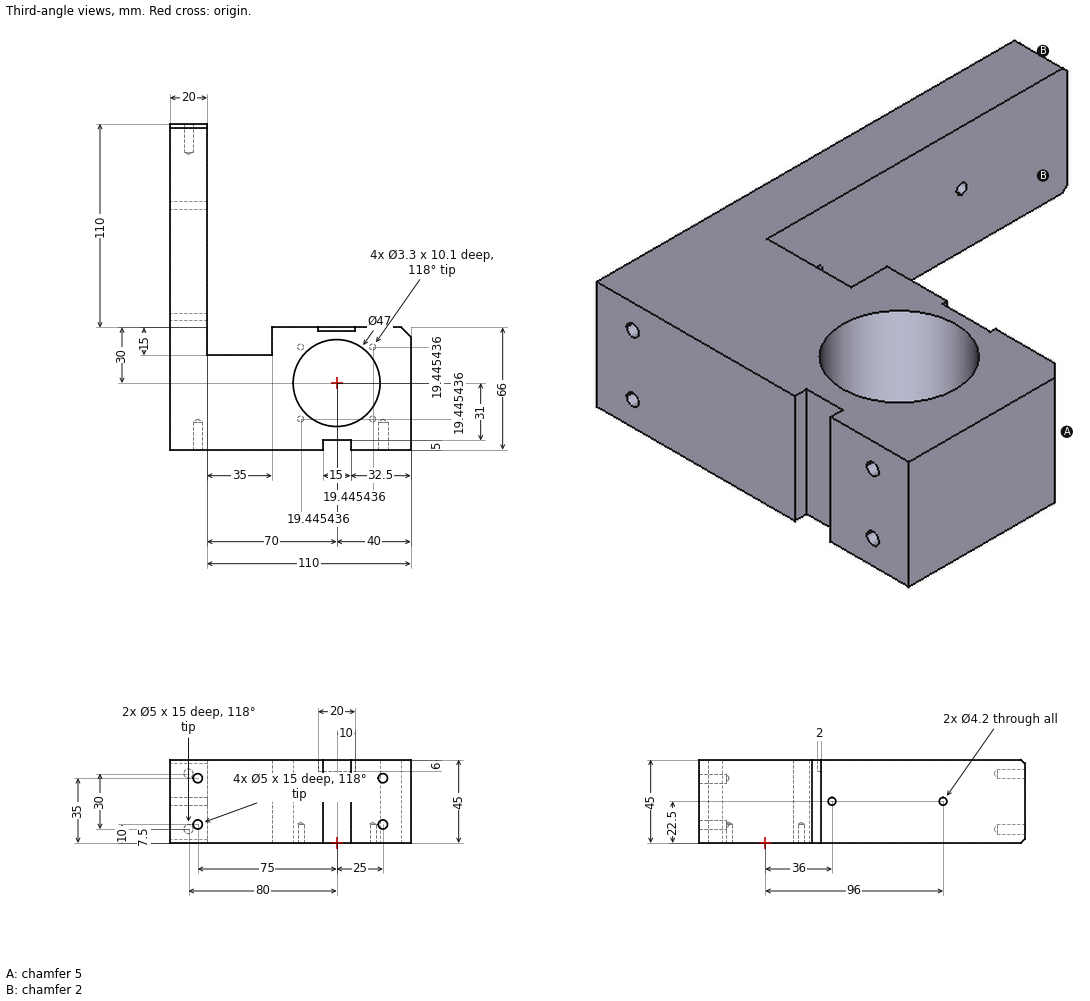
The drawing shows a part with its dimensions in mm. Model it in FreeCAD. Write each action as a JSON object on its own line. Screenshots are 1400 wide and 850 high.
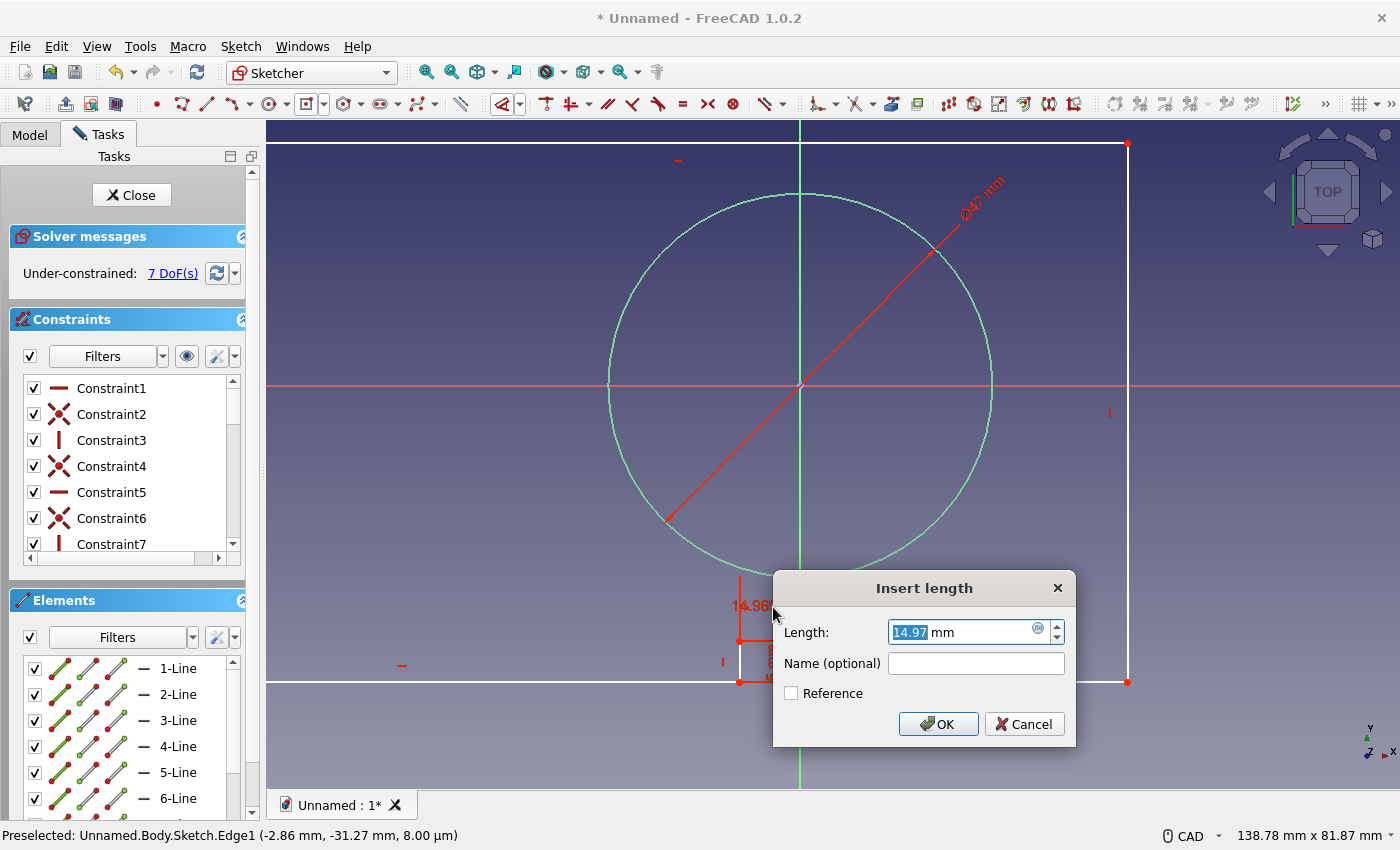
{"action": "type", "text": "15"}
{"action": "key", "text": "Return"}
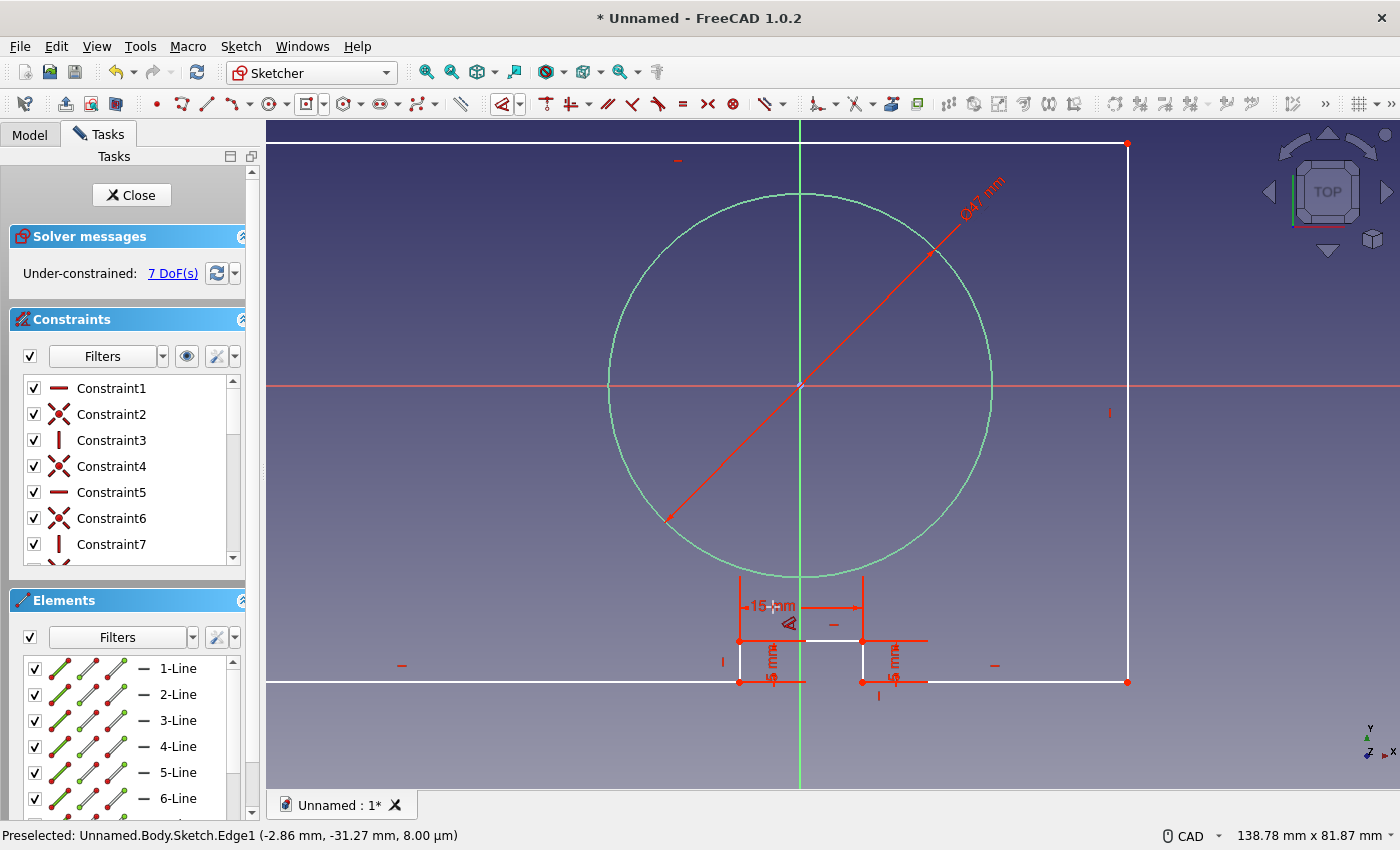
{"action": "left_click", "coordinate": [1128, 520]}
{"action": "left_click", "coordinate": [1162, 415]}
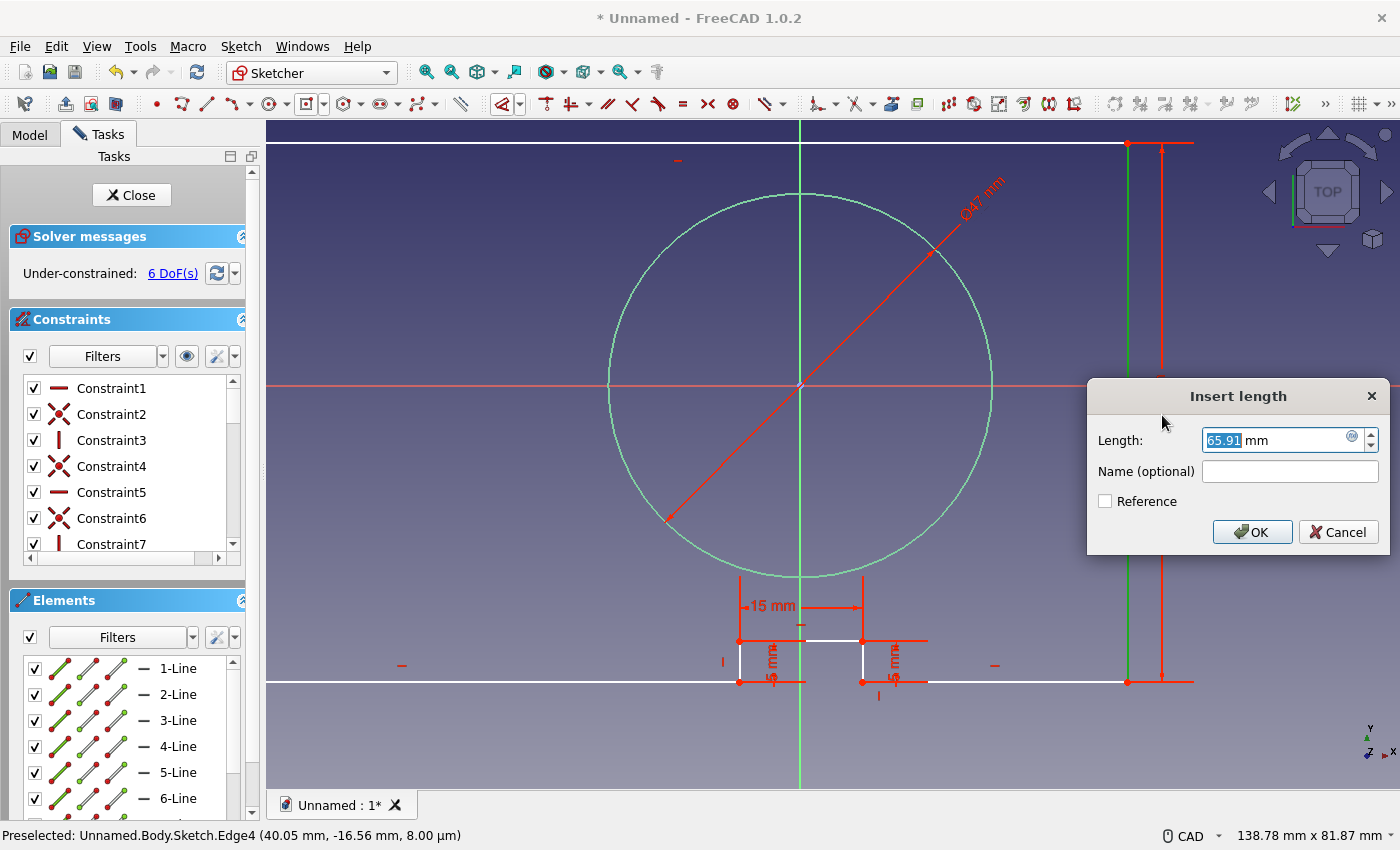
{"action": "type", "text": "66"}
{"action": "key", "text": "Return"}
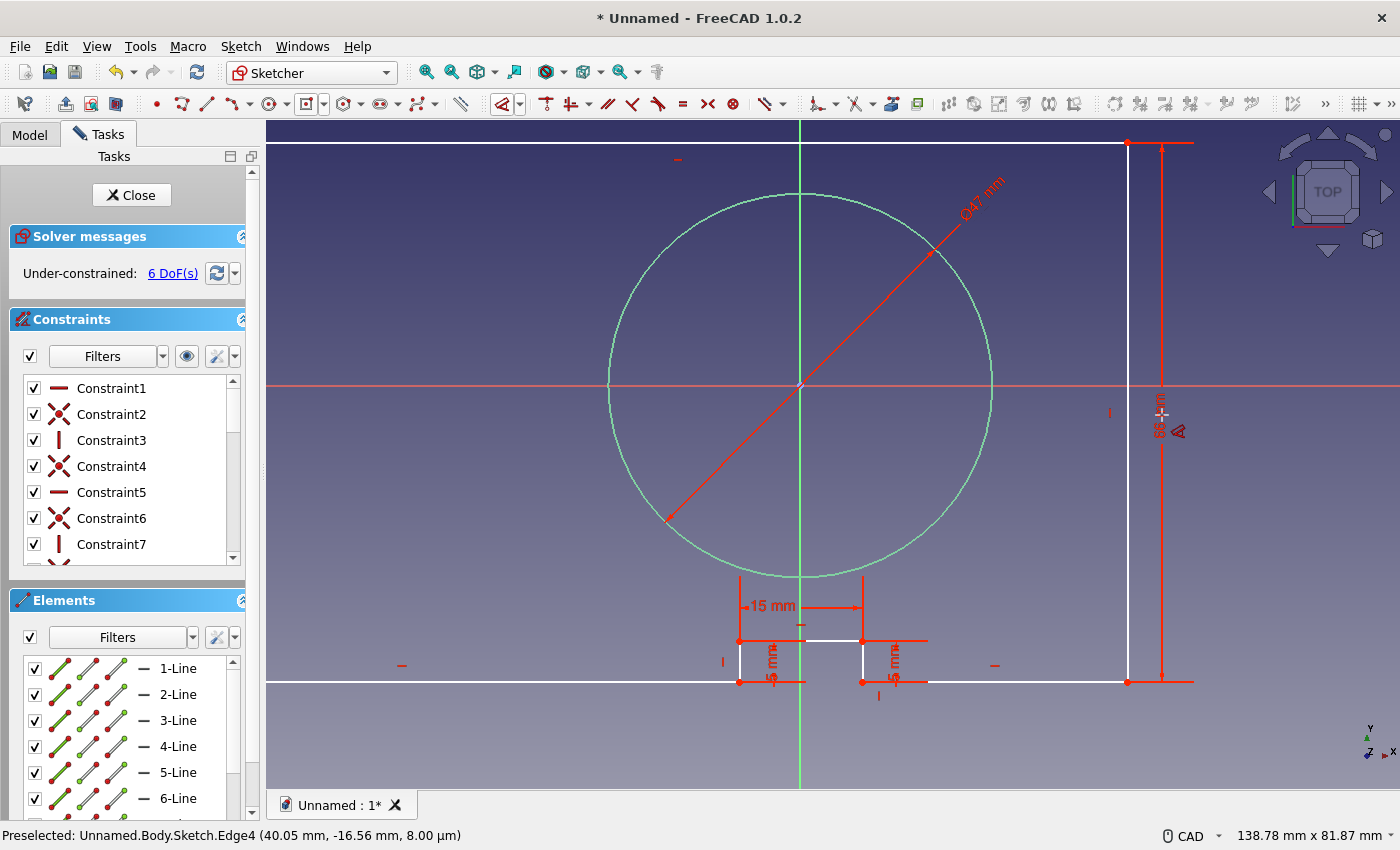
{"action": "scroll", "coordinate": [837, 667], "scroll_direction": "down", "scroll_amount": 6}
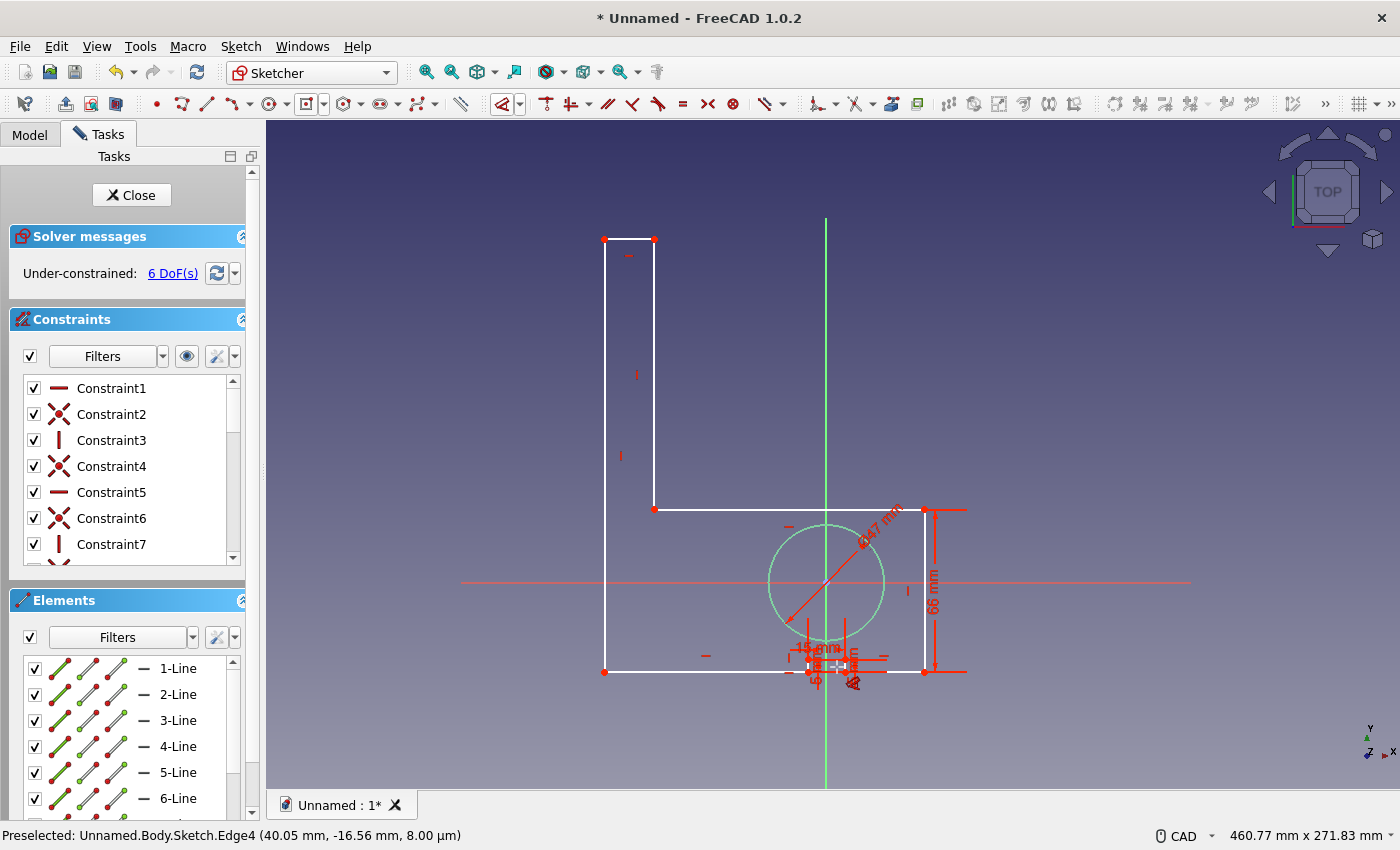
{"action": "left_click", "coordinate": [639, 239]}
{"action": "left_click", "coordinate": [630, 205]}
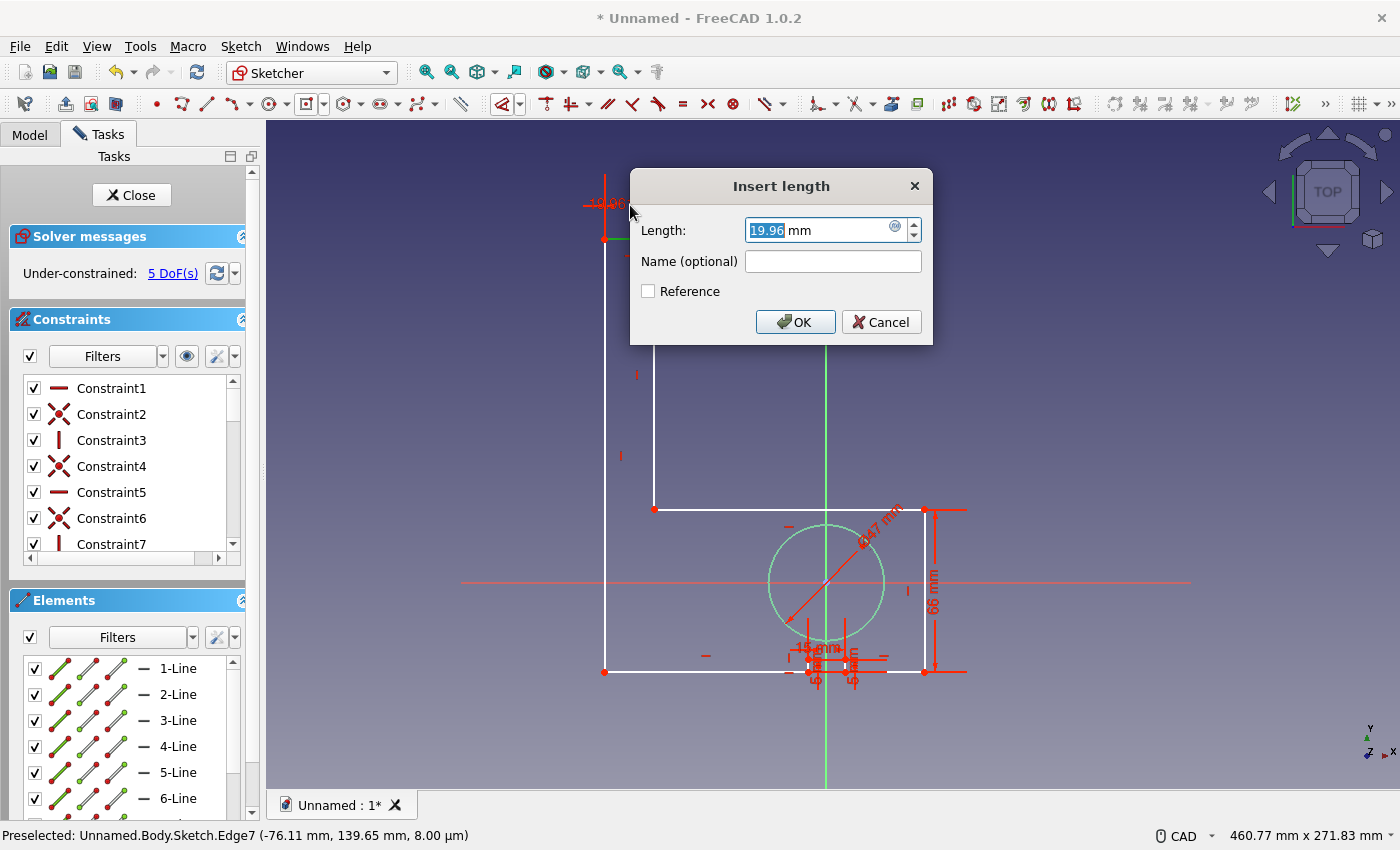
{"action": "type", "text": "20"}
{"action": "key", "text": "Return"}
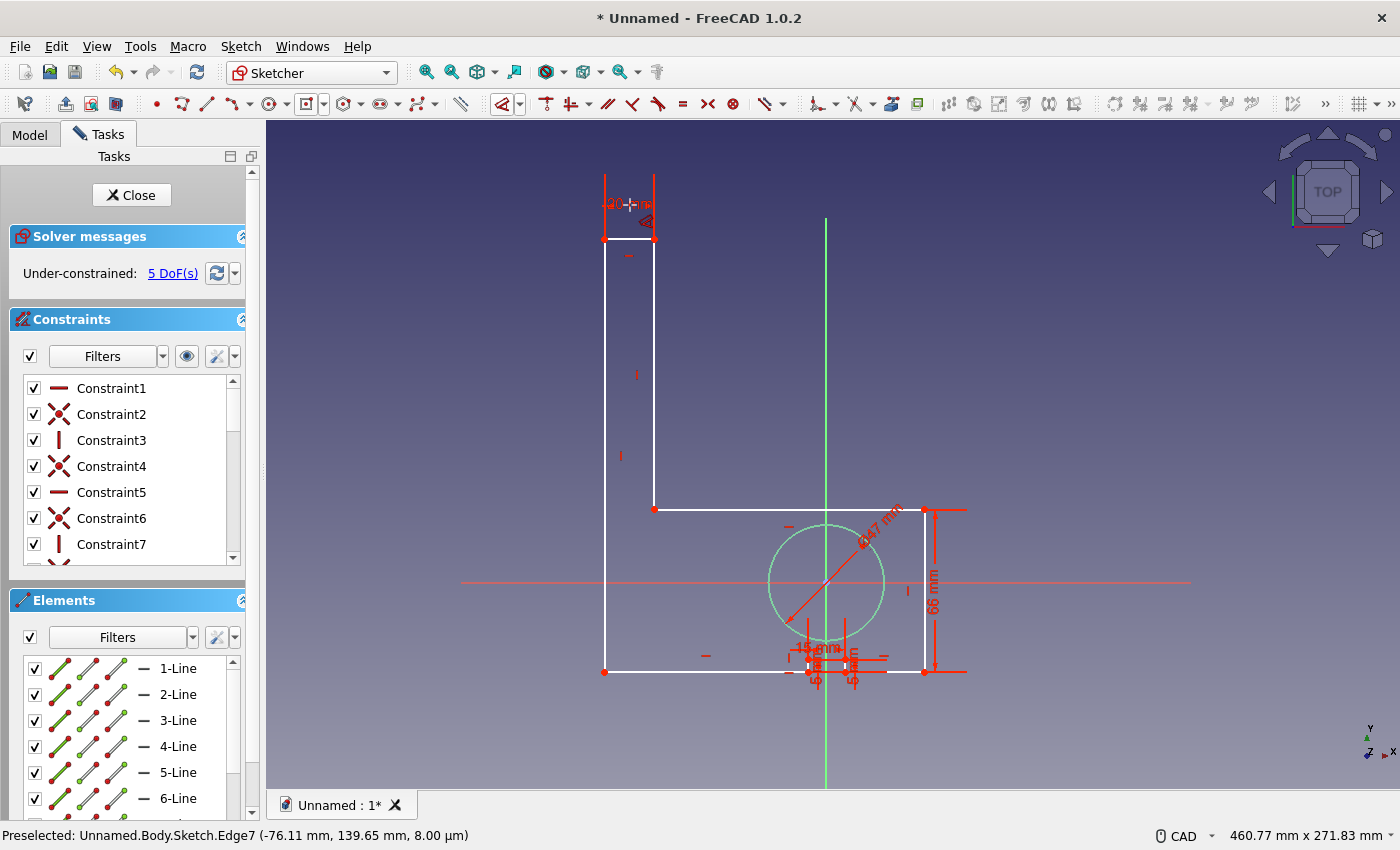
{"action": "left_click", "coordinate": [844, 510]}
{"action": "left_click", "coordinate": [727, 544]}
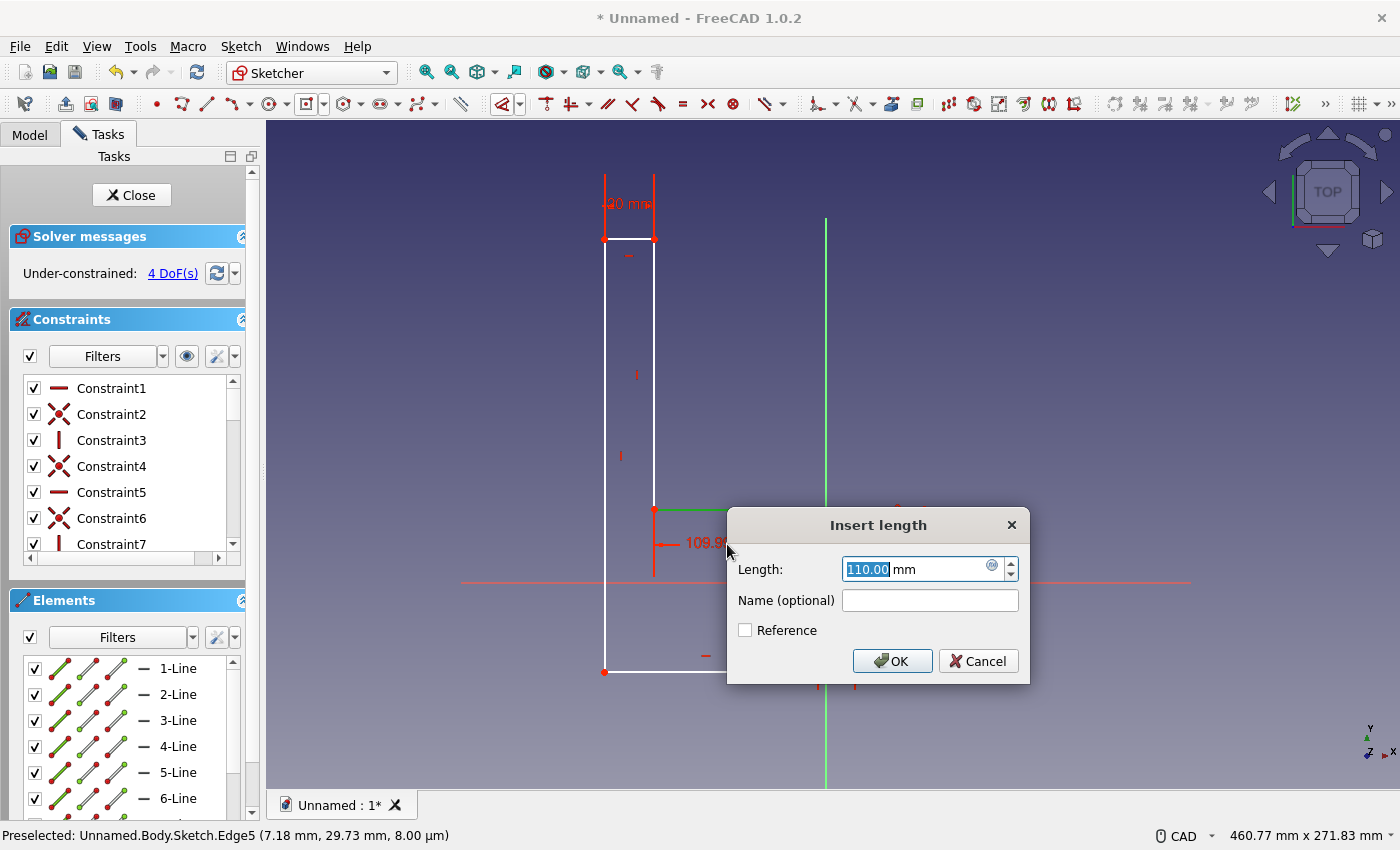
{"action": "type", "text": "110"}
{"action": "key", "text": "Return"}